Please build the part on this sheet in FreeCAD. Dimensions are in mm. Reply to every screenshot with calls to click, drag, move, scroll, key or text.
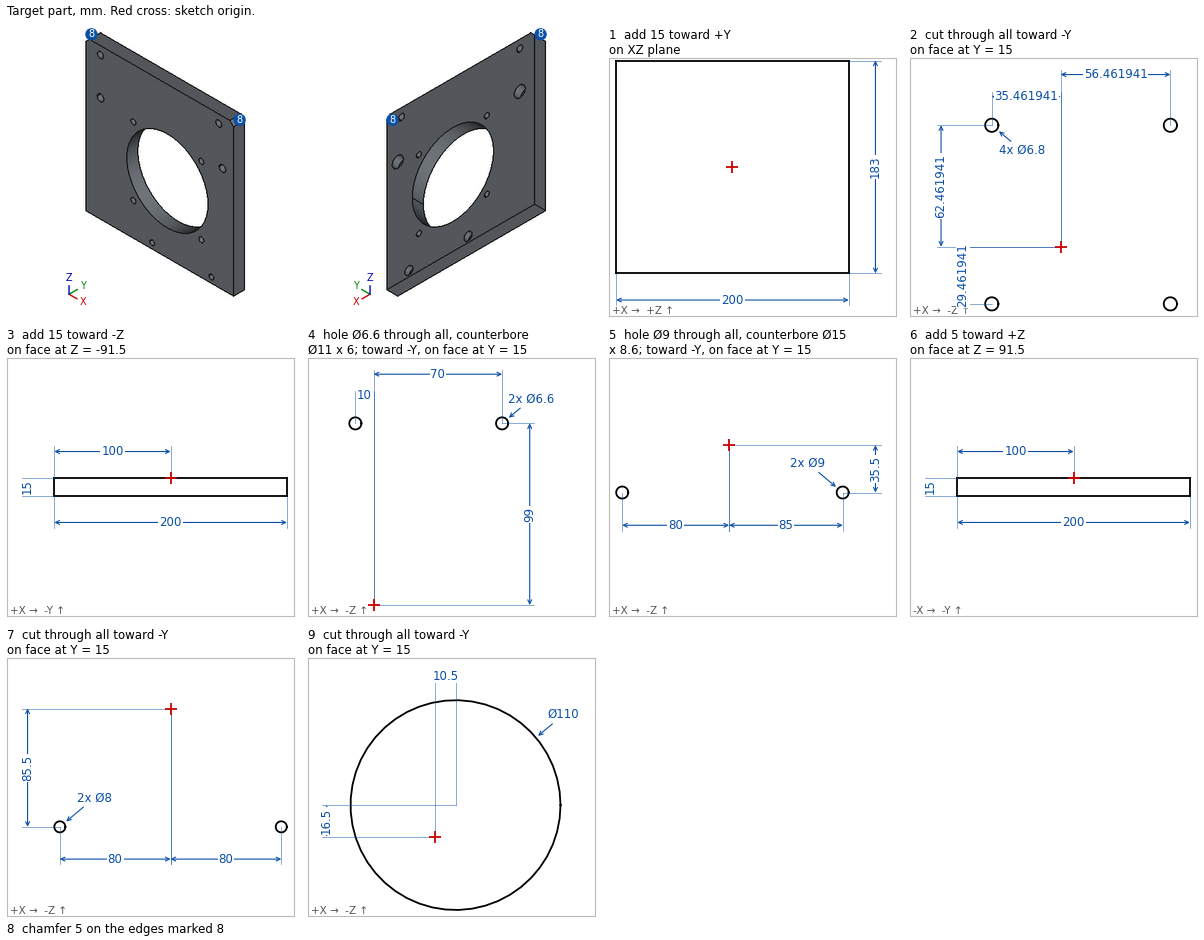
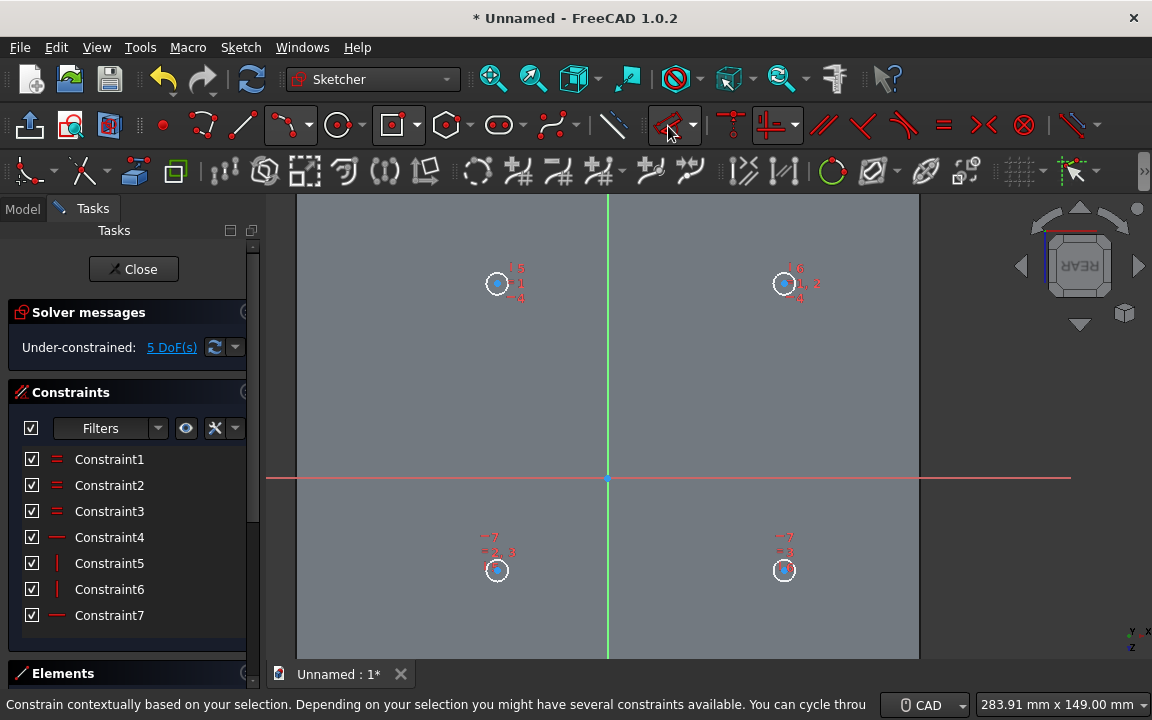
scroll(505, 276, up, 4)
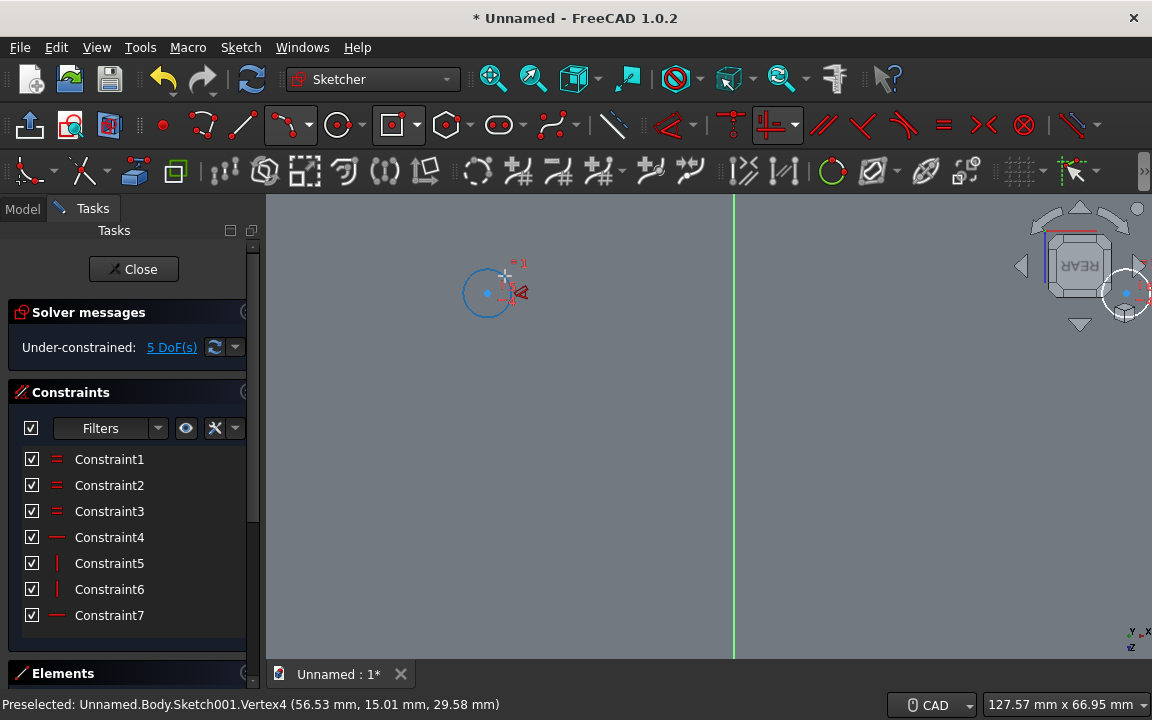
click(504, 276)
click(526, 253)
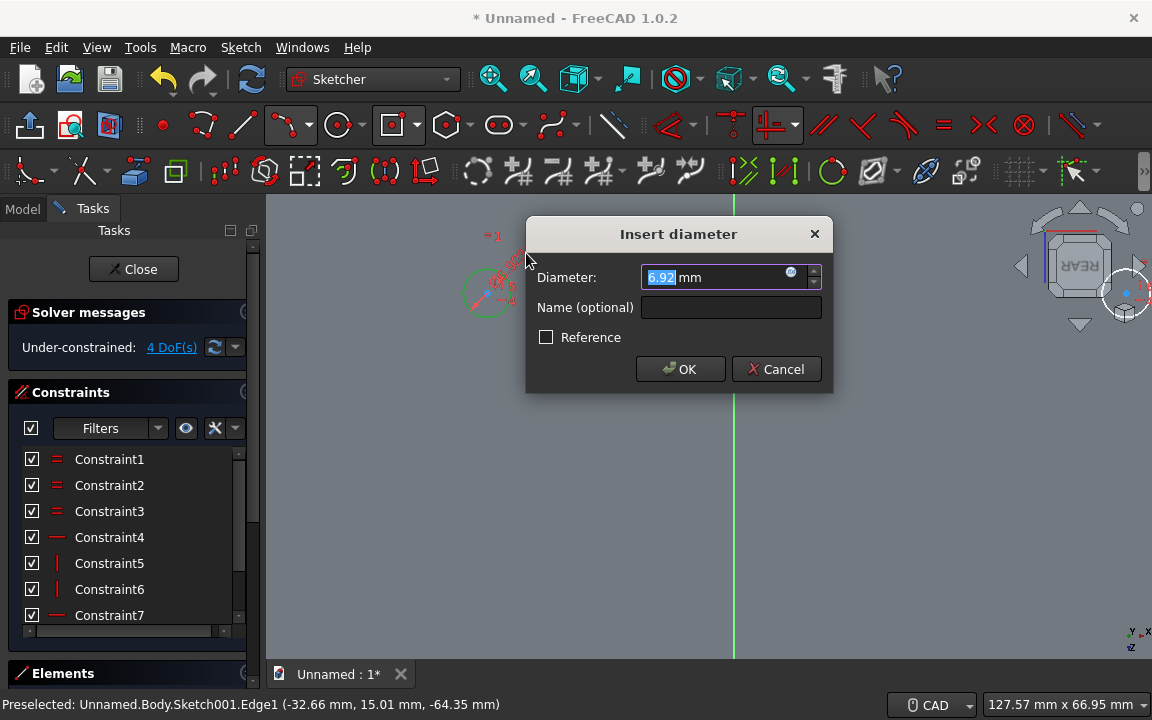
text(6.8)
key(Return)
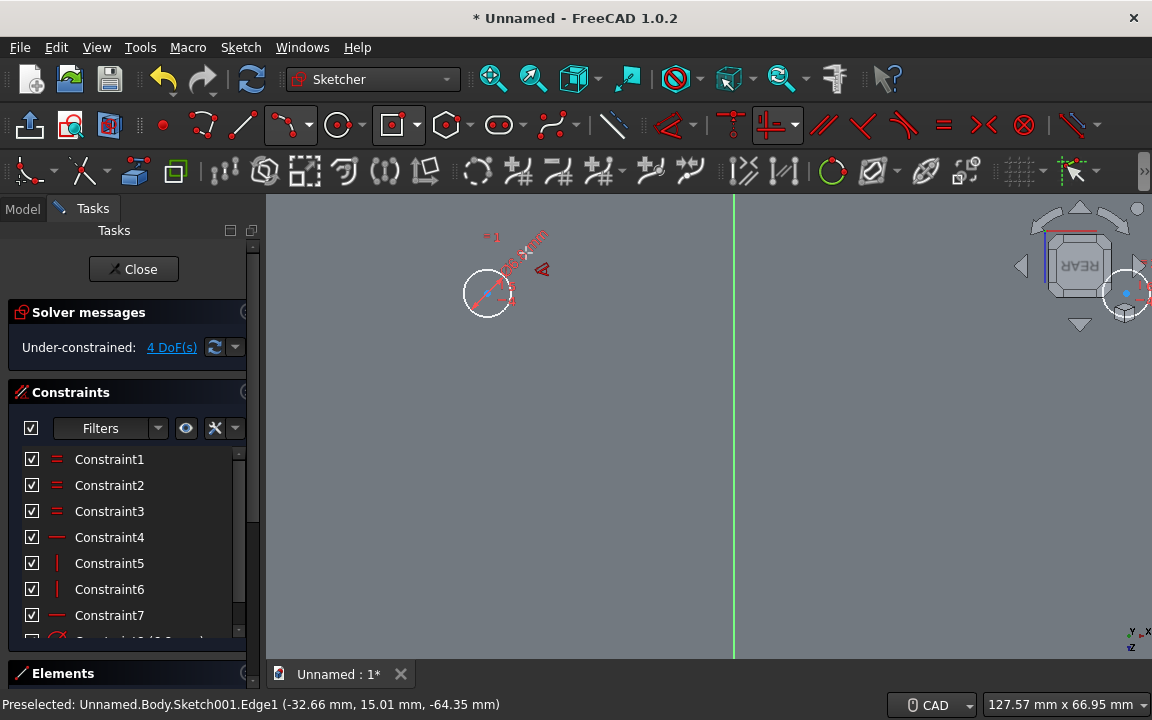
click(487, 293)
click(611, 259)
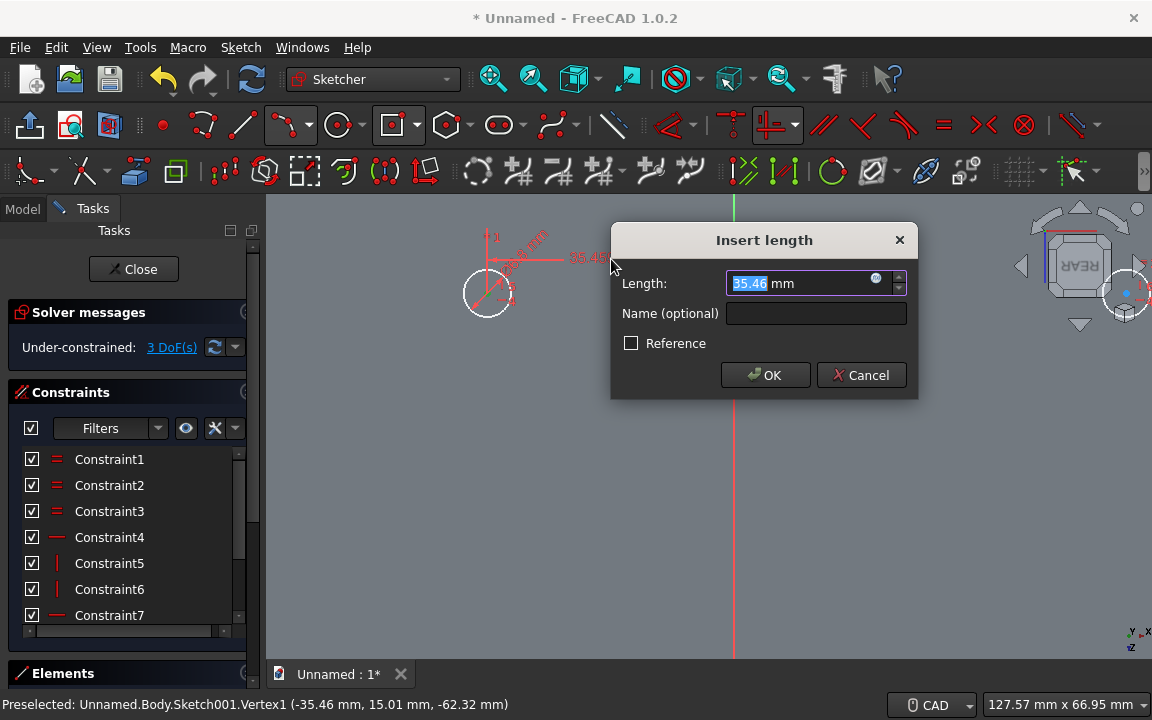
text(35.461941)
key(Return)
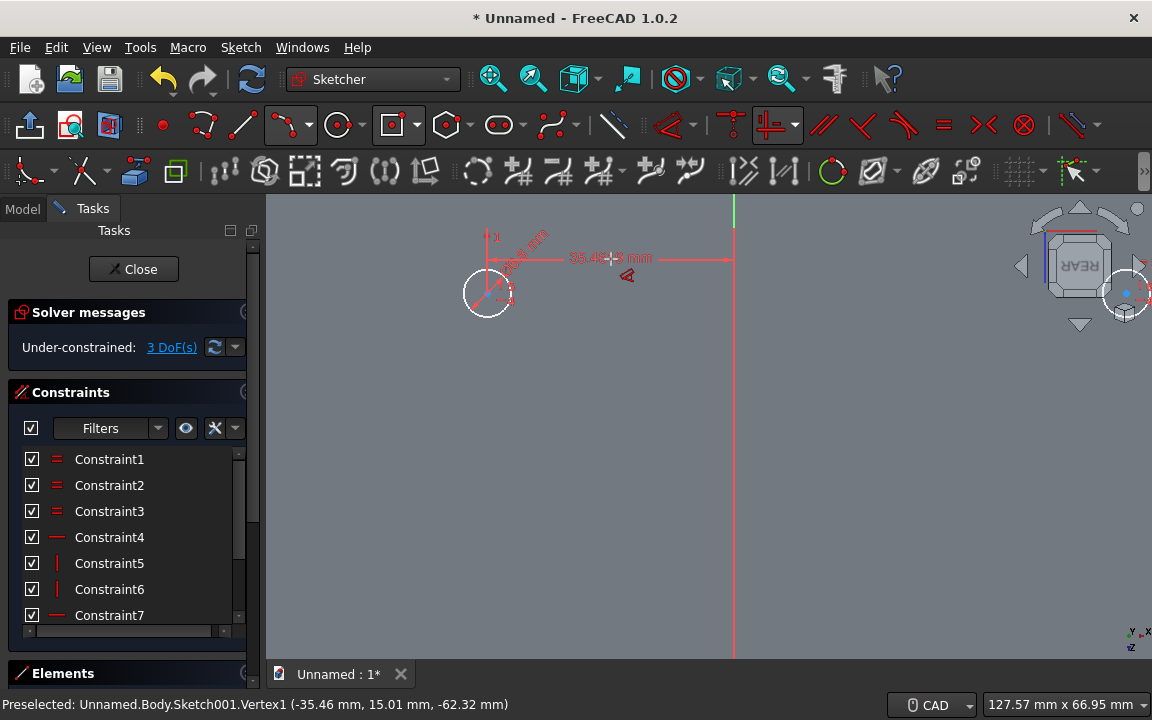
click(487, 293)
click(453, 462)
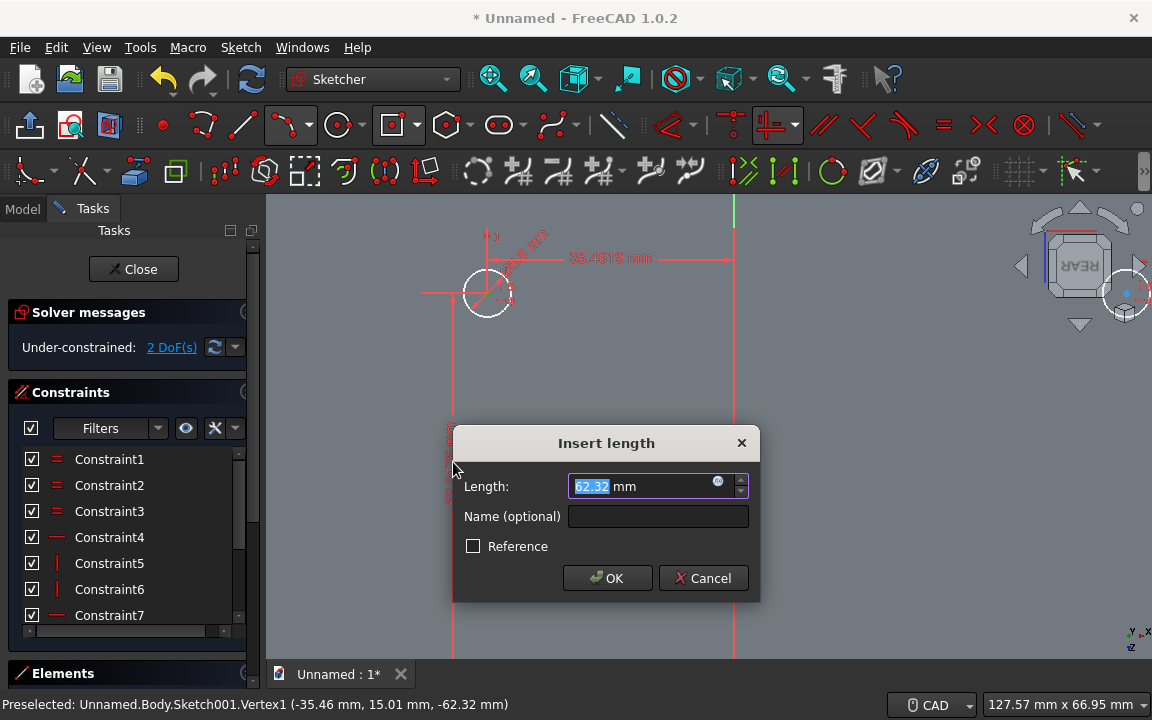
text(62.461941)
key(Return)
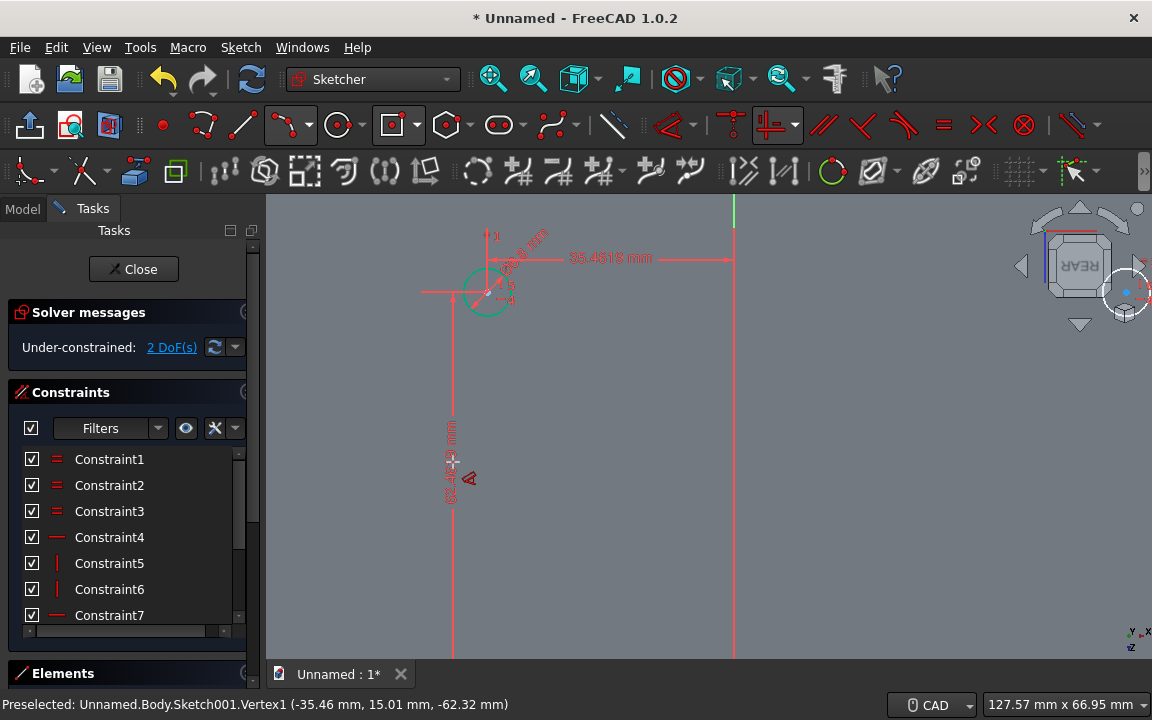
scroll(505, 276, down, 4)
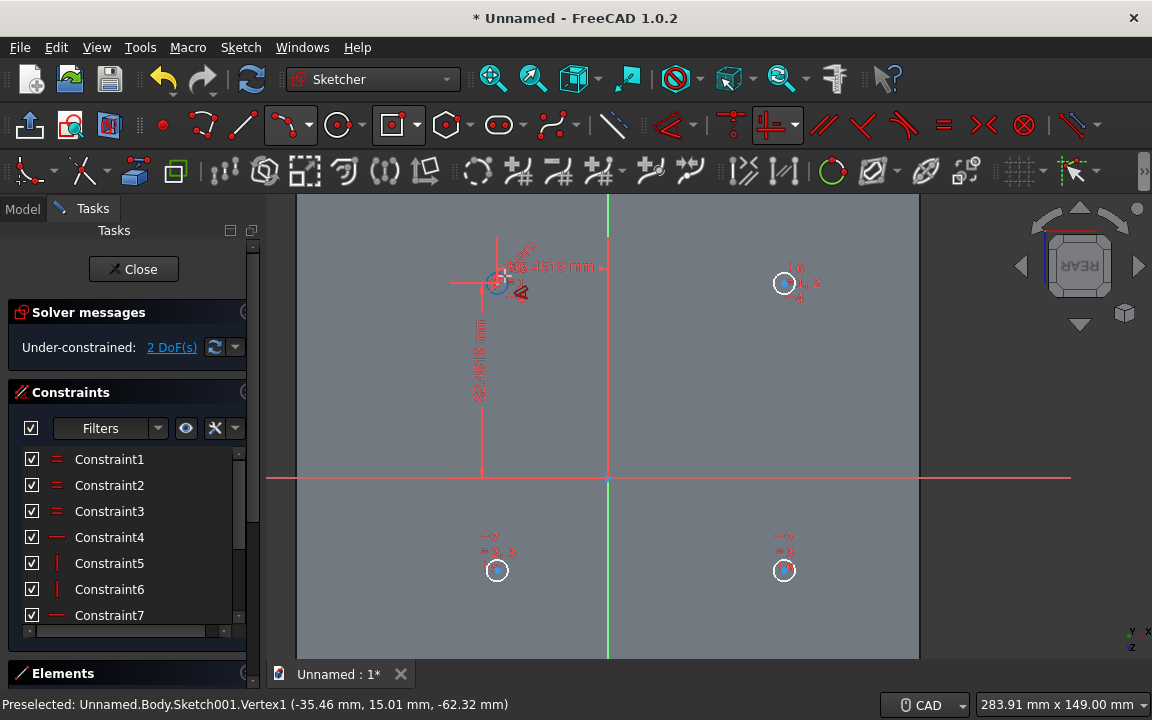
click(784, 283)
click(696, 249)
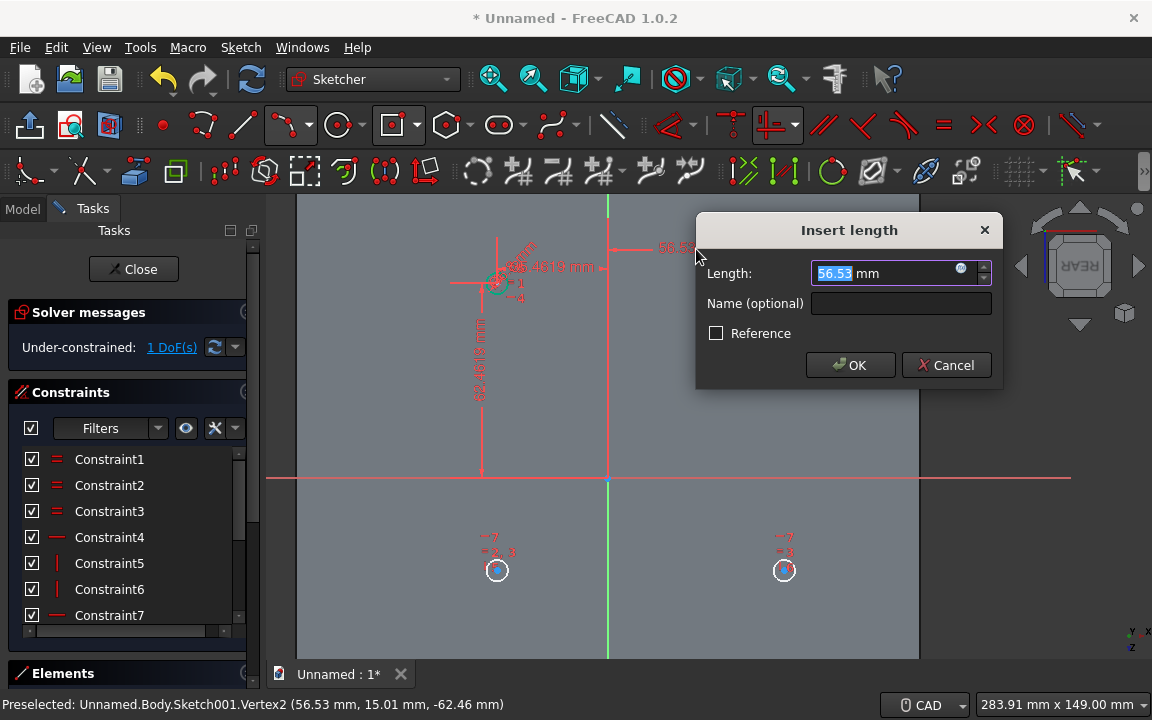
text(56.461941)
key(Return)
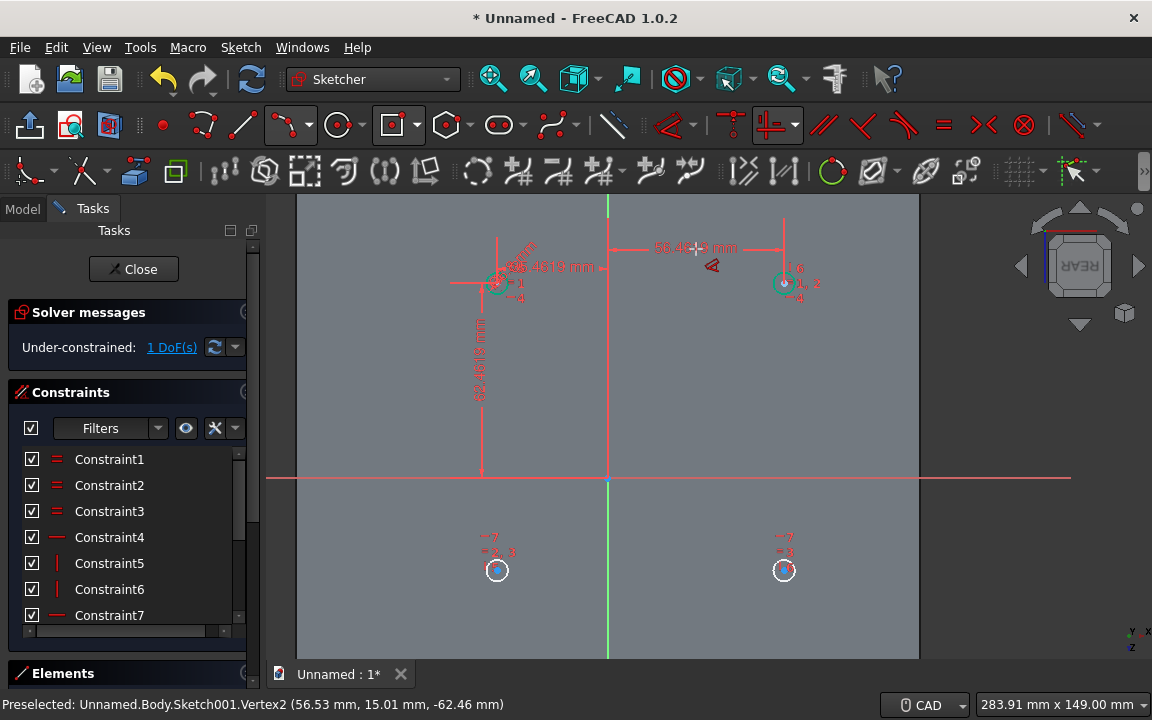
click(497, 571)
click(463, 525)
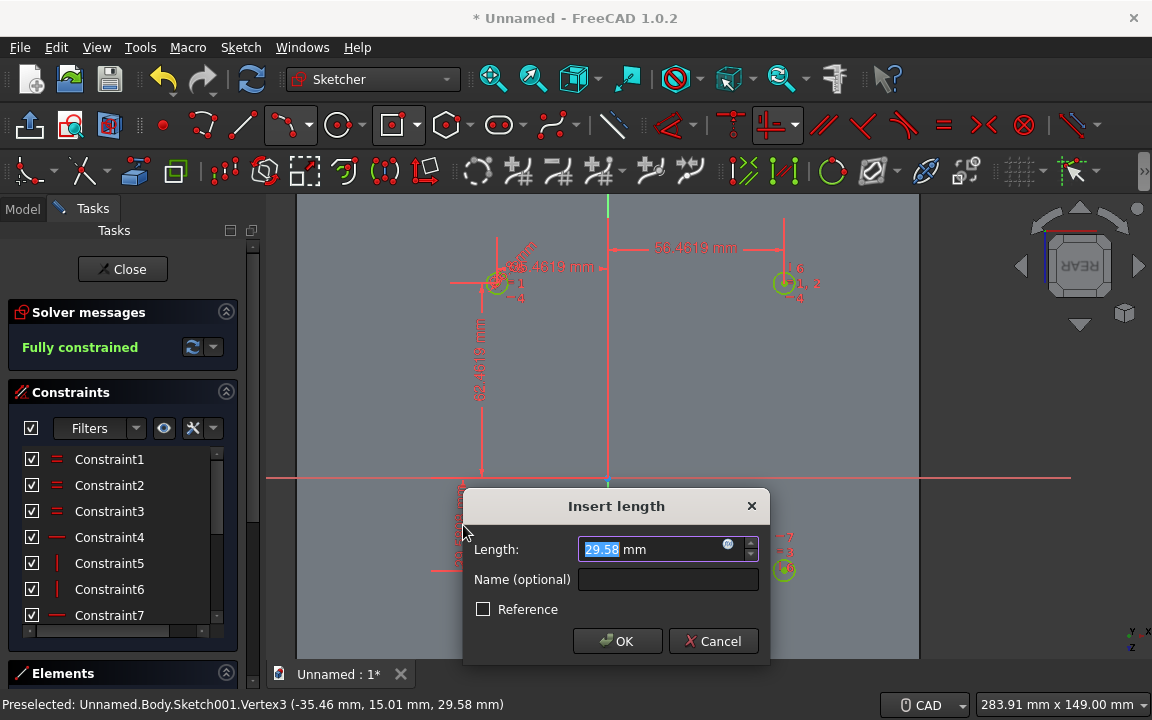
text(29.461941)
key(Return)
key(Escape)